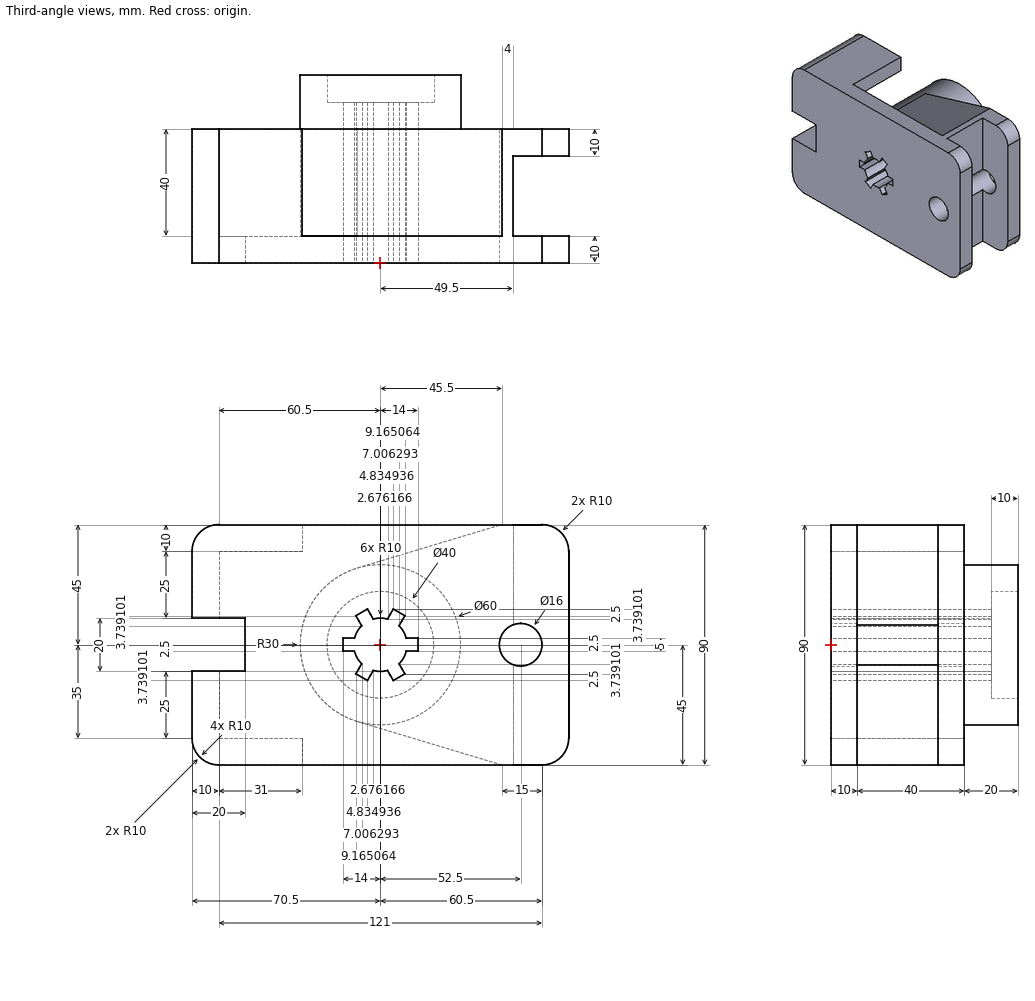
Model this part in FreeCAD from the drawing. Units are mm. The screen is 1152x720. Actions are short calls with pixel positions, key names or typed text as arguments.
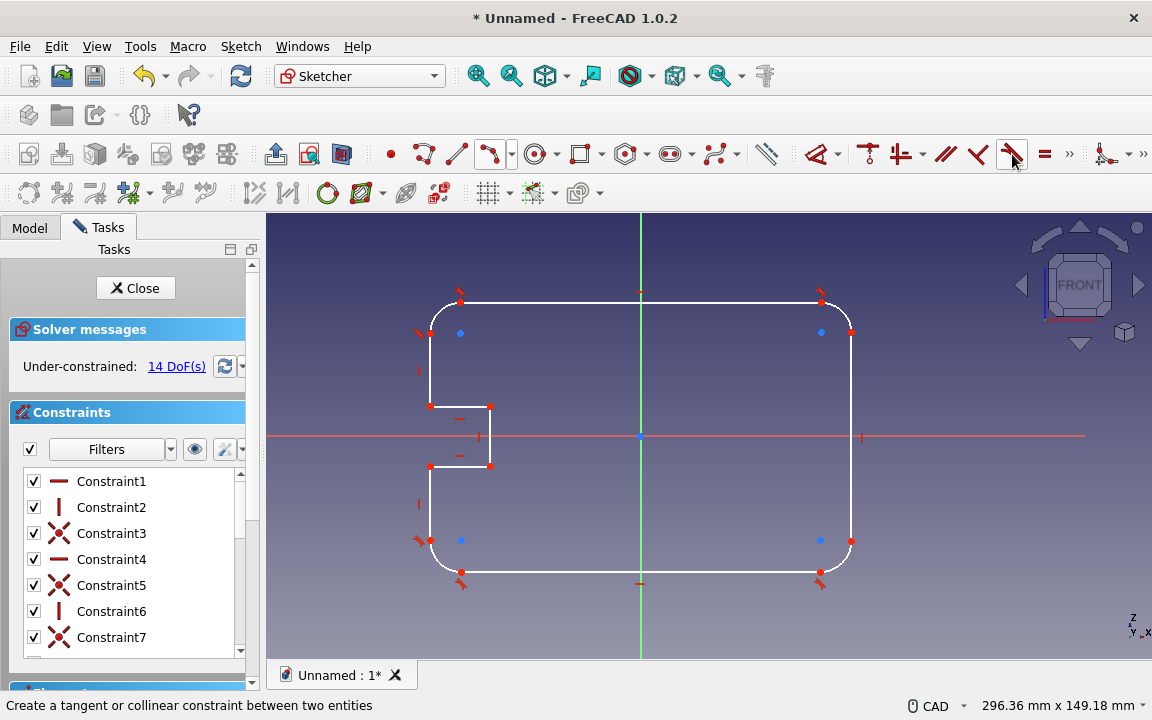
click(851, 396)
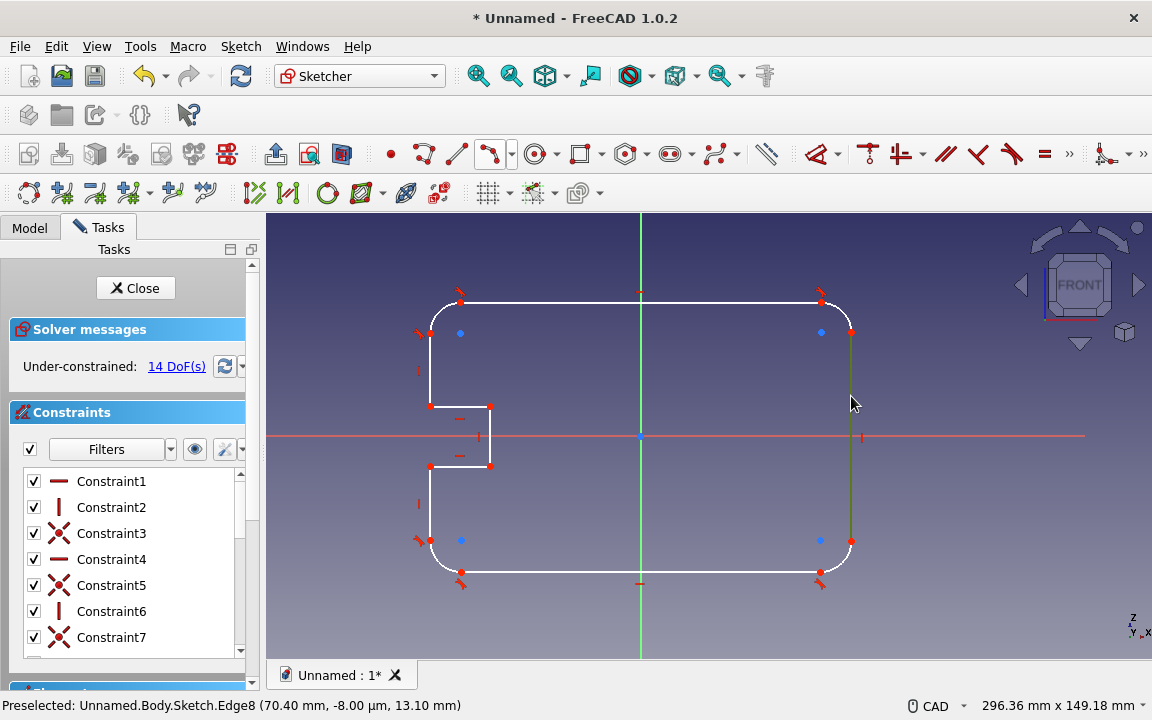
click(848, 319)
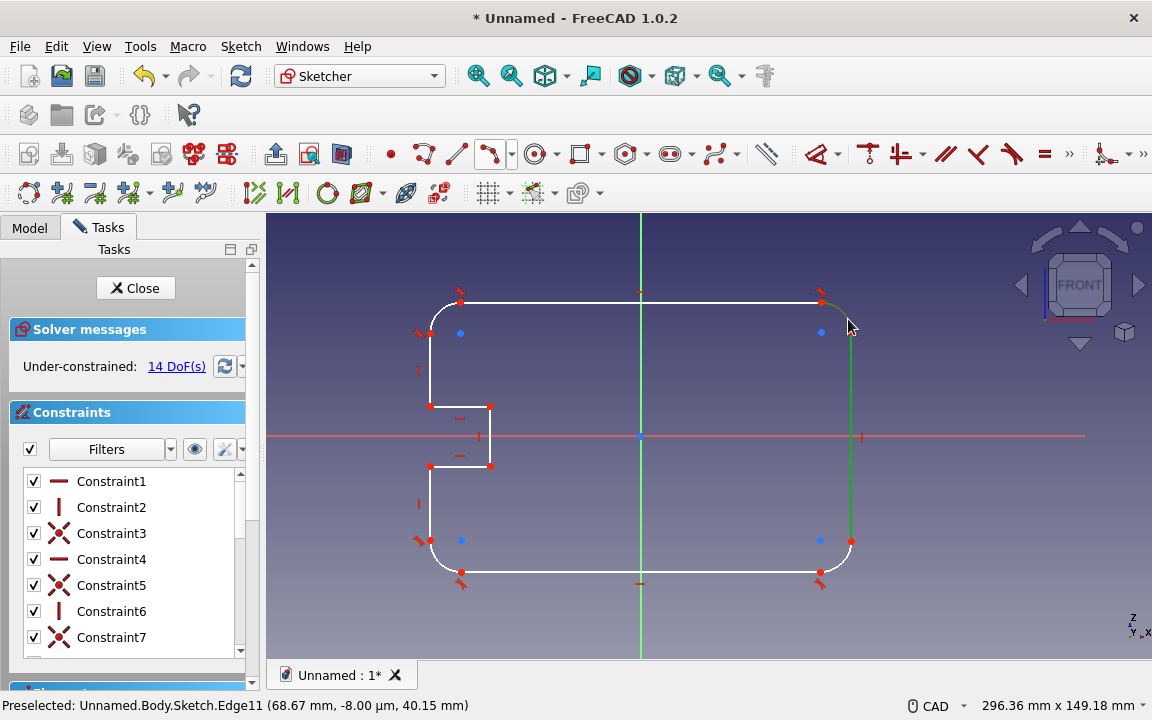
click(1012, 154)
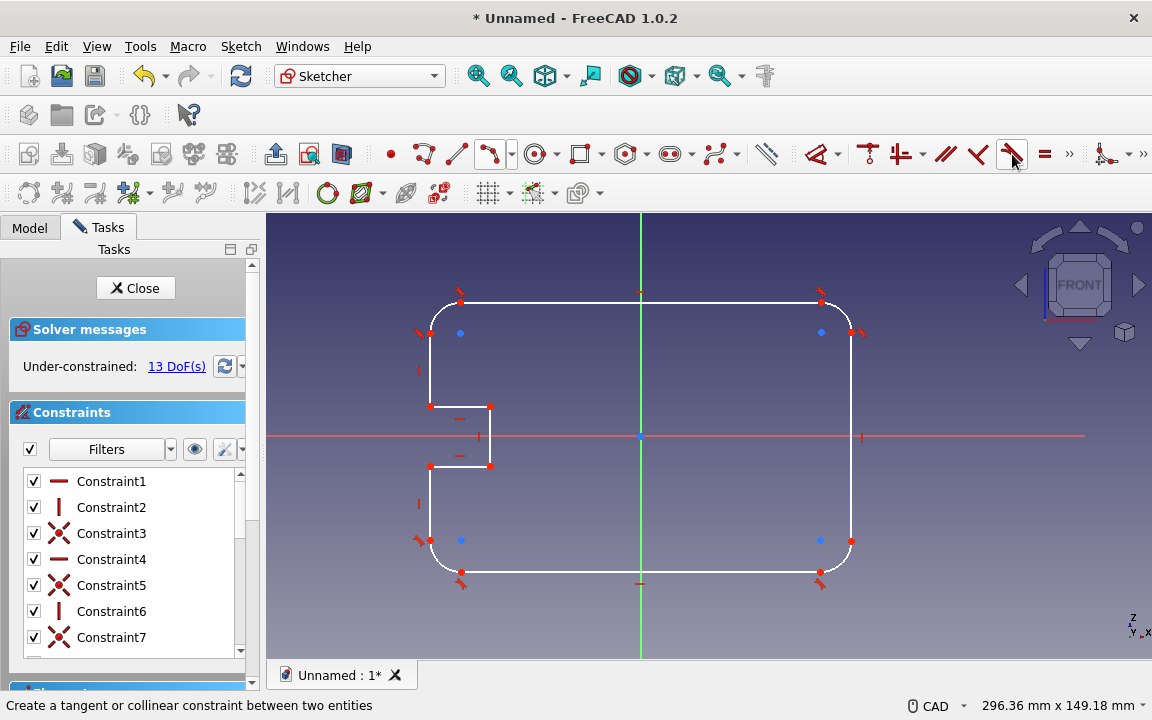
click(851, 396)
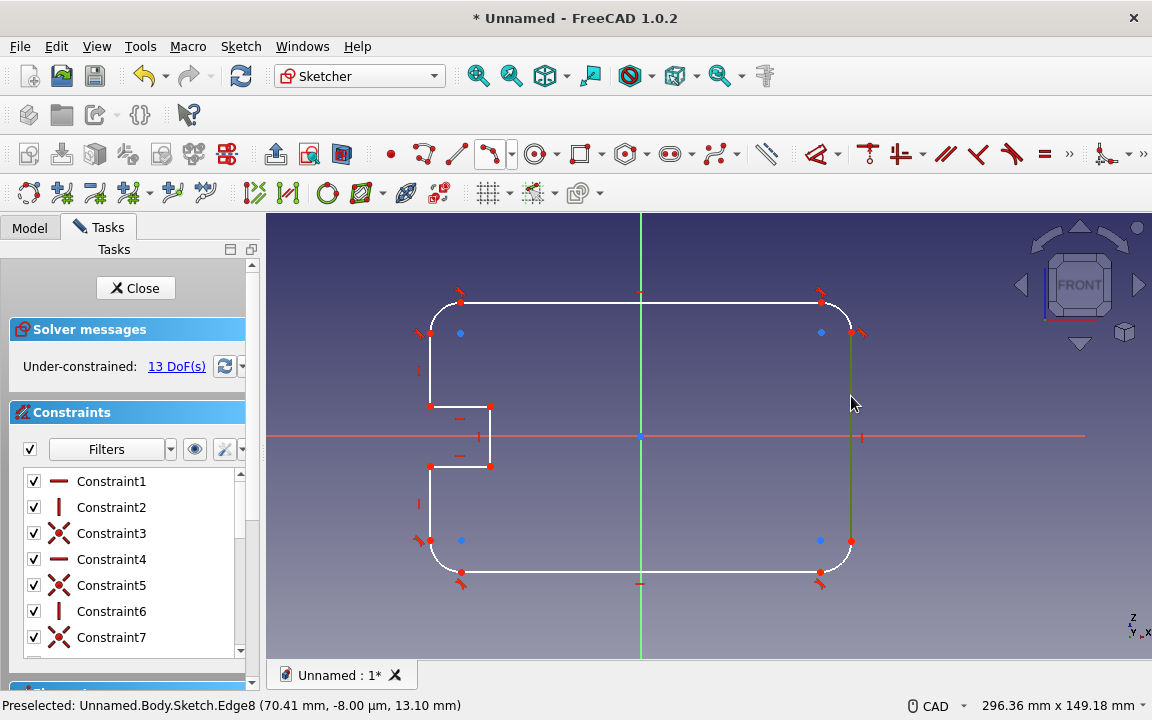
click(834, 569)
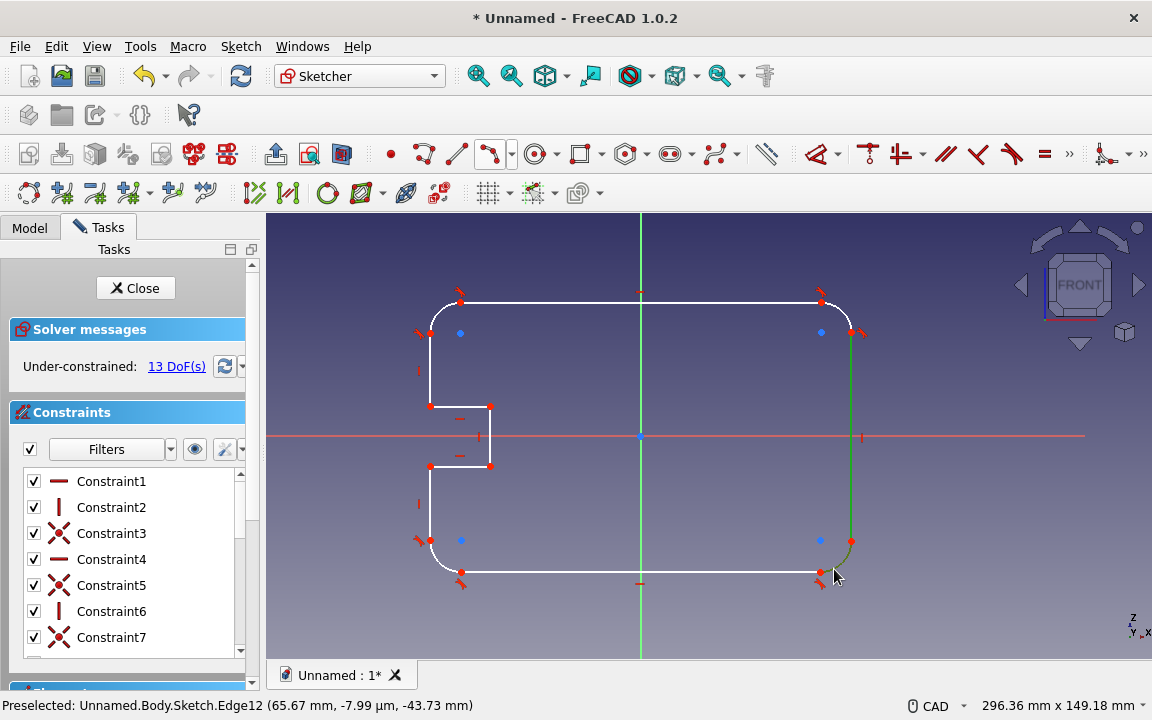
click(1012, 154)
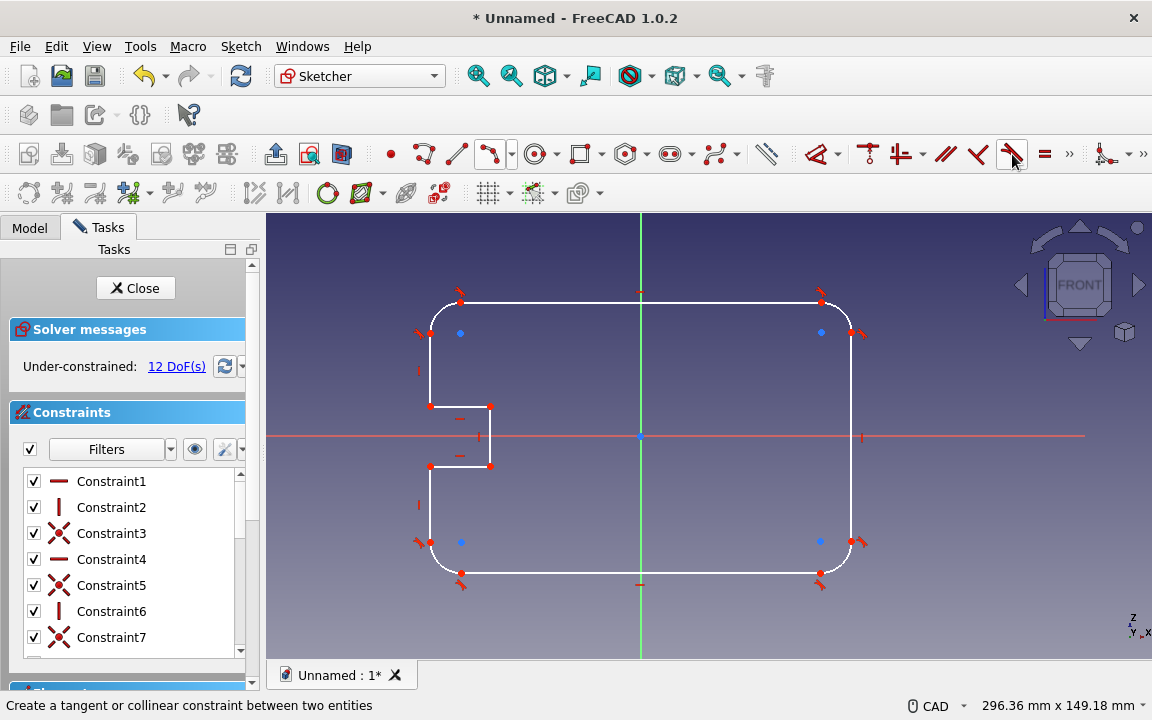
click(434, 556)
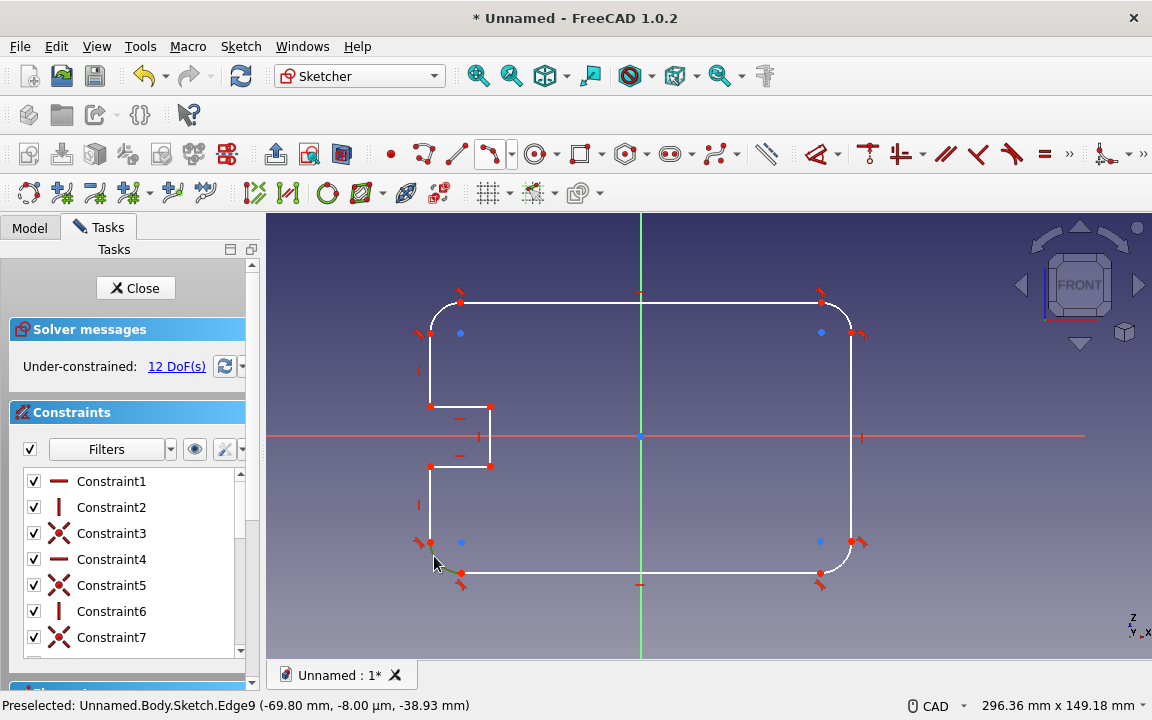
click(447, 306)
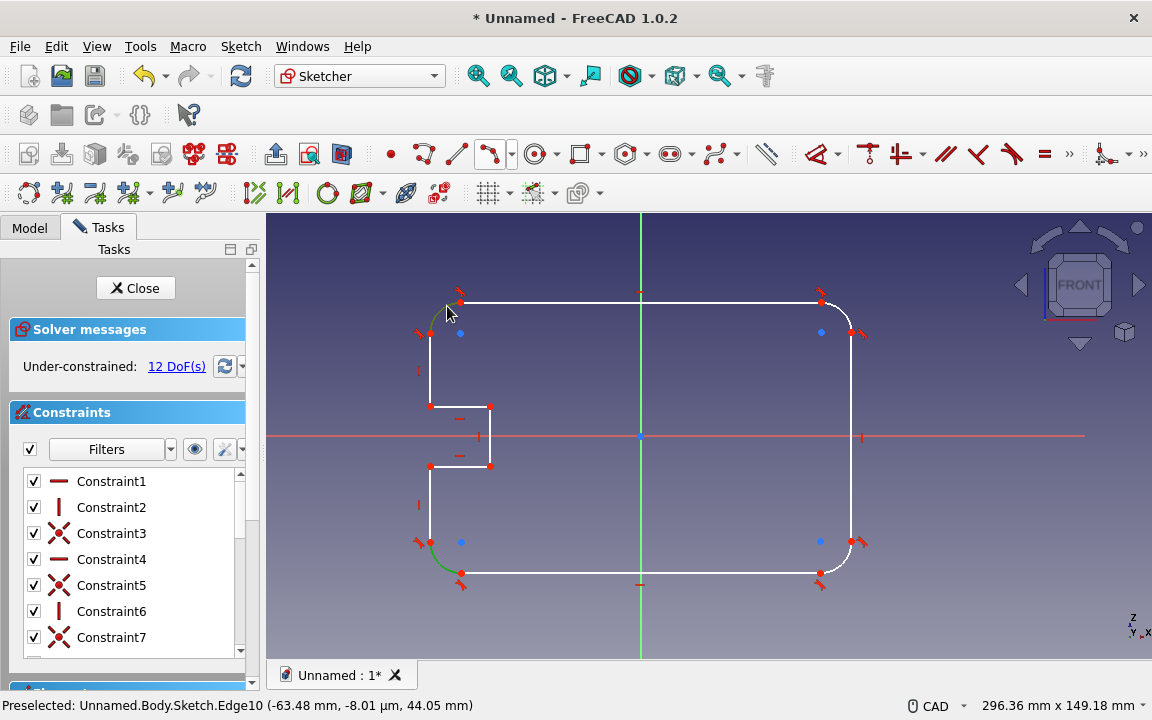
click(848, 319)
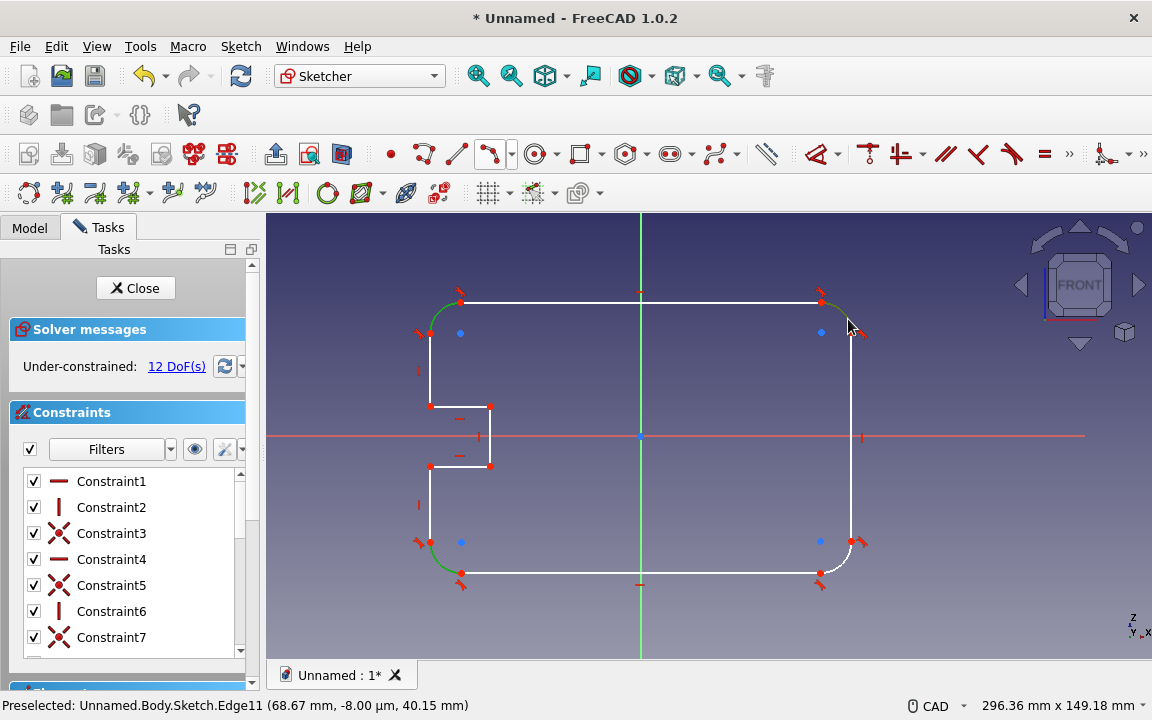
click(834, 570)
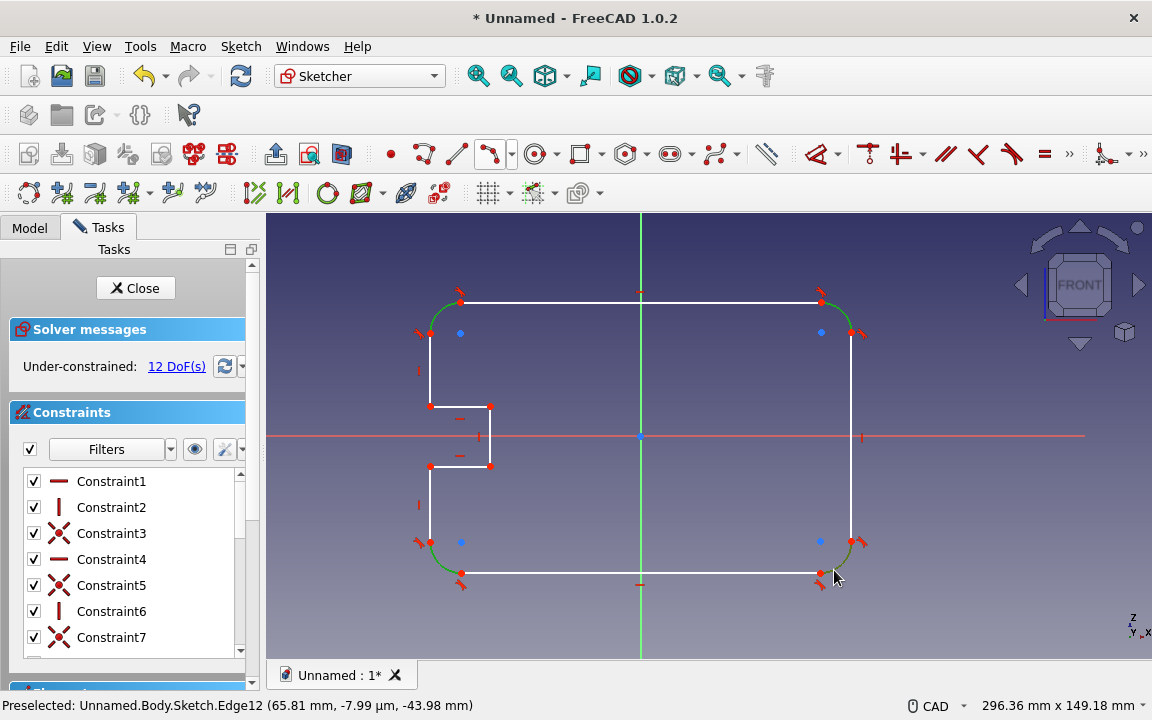
click(1045, 154)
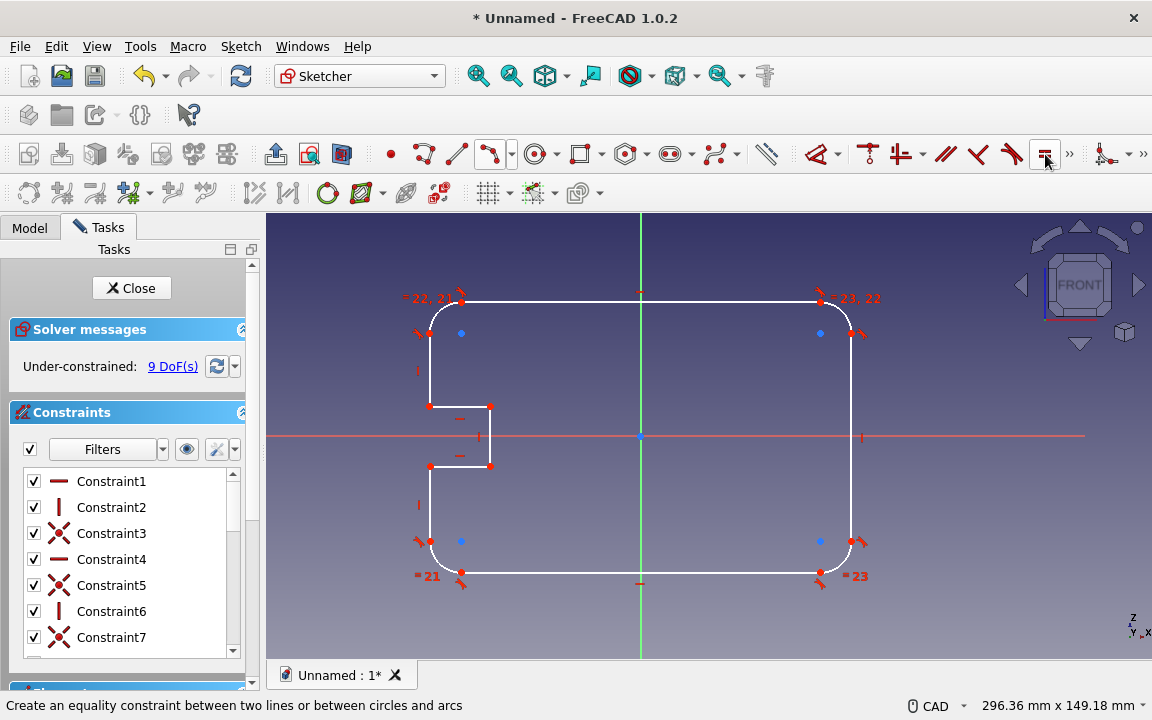
scroll(434, 556, up, 2)